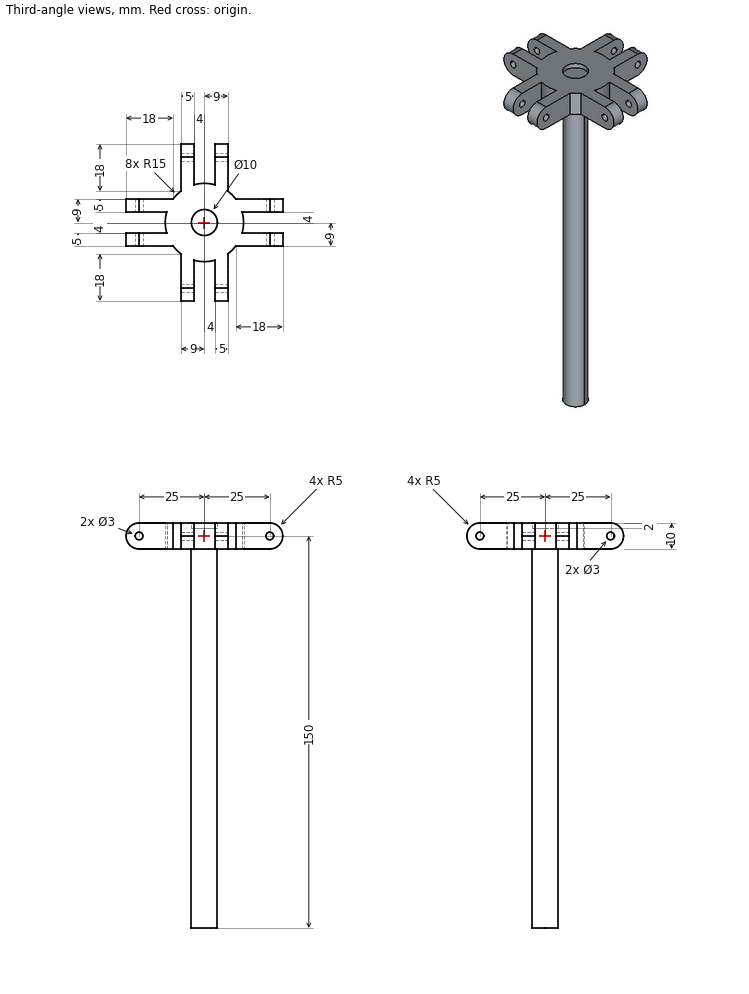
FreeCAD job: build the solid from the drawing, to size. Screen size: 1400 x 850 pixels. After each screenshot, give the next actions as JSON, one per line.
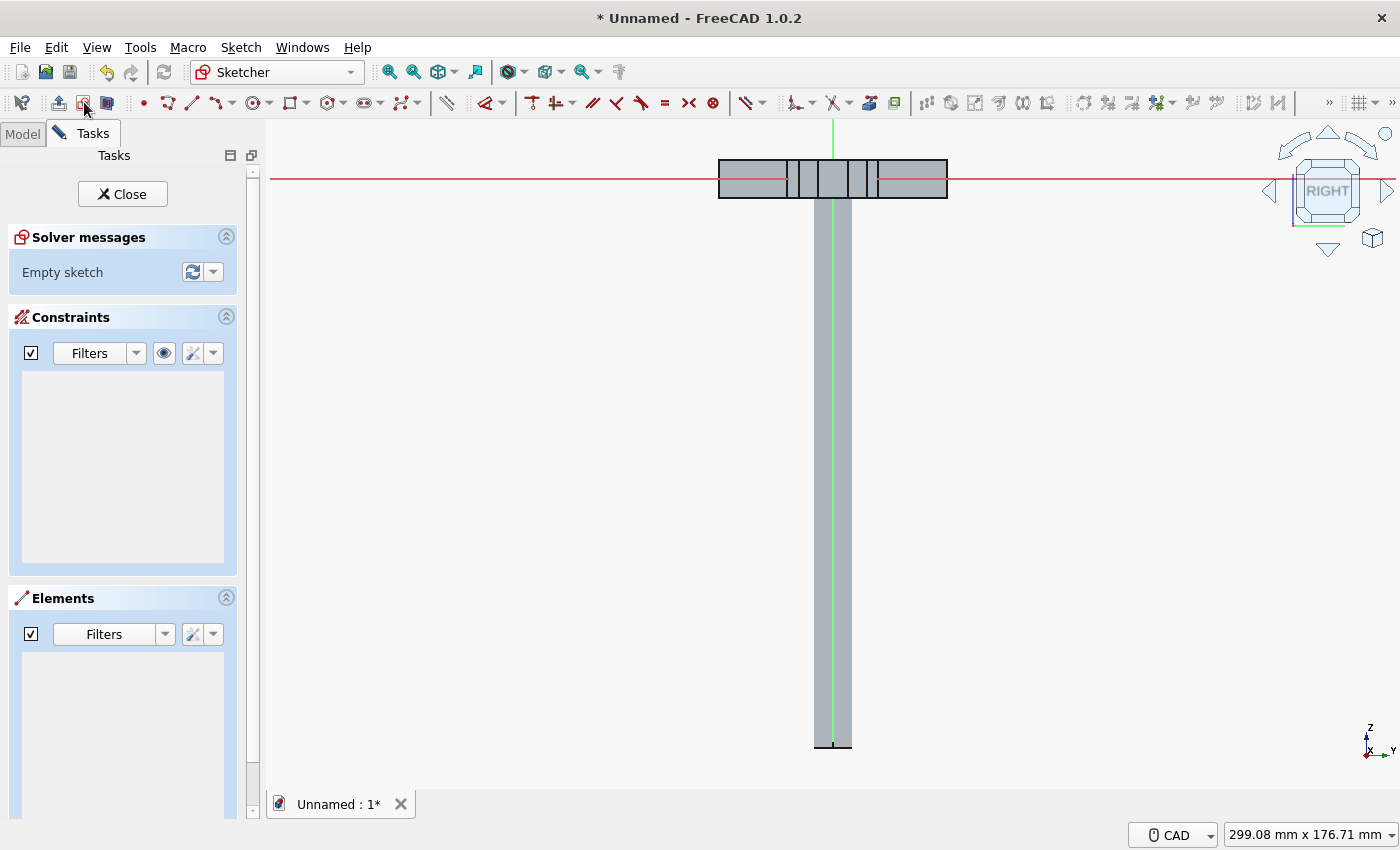
{"action": "scroll", "coordinate": [873, 147], "scroll_direction": "up", "scroll_amount": 5}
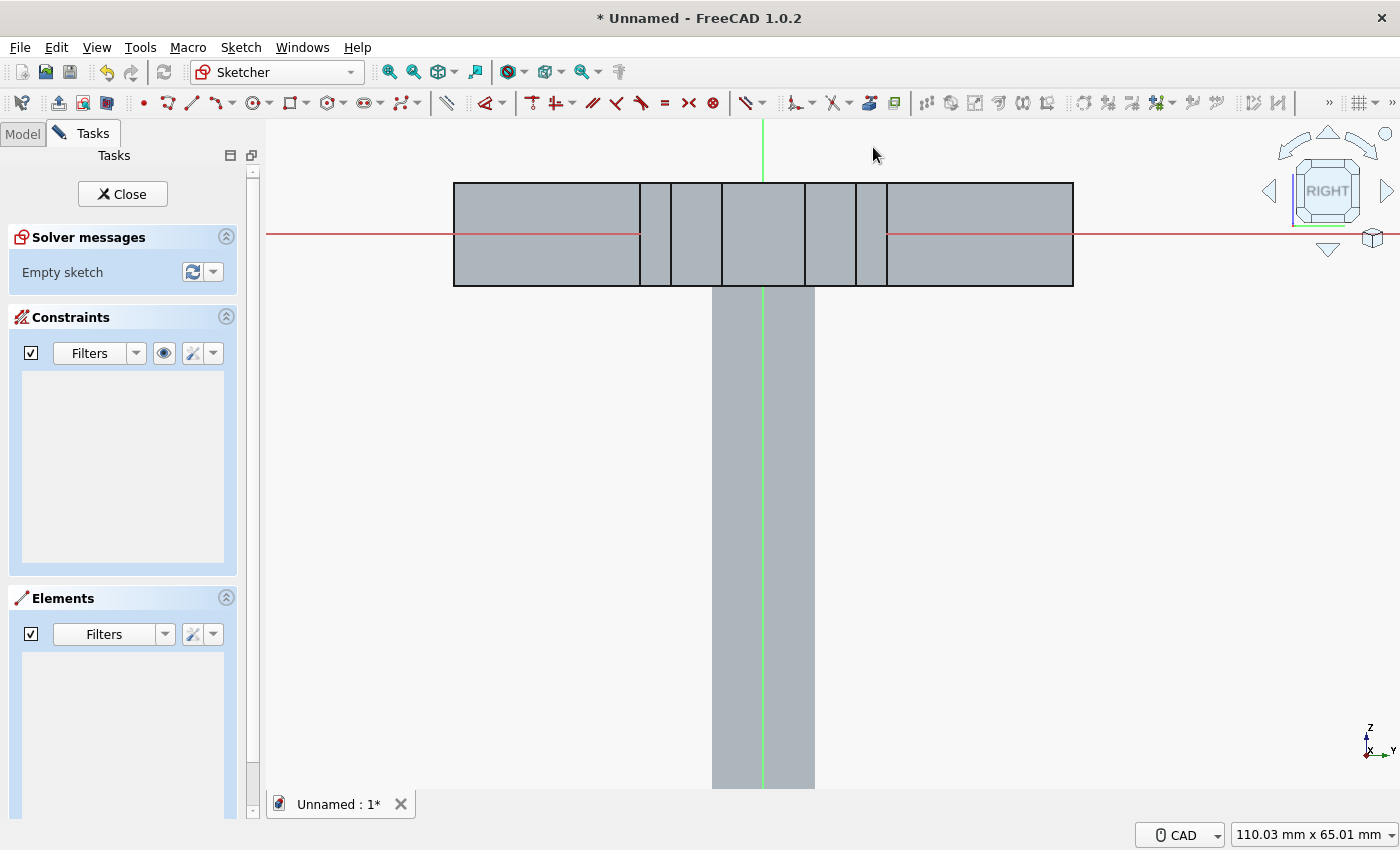
{"action": "left_click", "coordinate": [168, 104]}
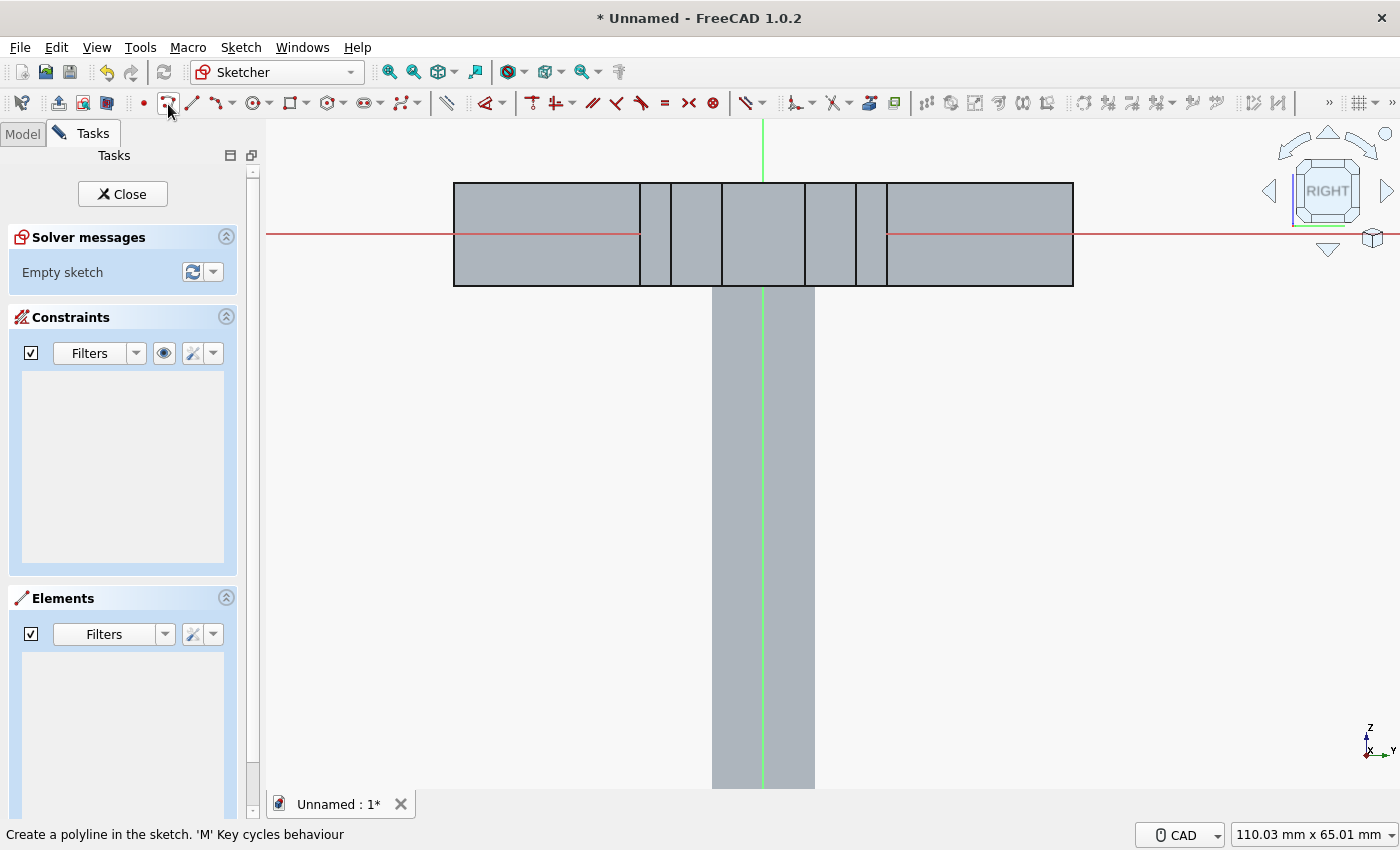
{"action": "left_click", "coordinate": [506, 183]}
{"action": "left_click", "coordinate": [454, 183]}
{"action": "left_click", "coordinate": [454, 234]}
{"action": "right_click", "coordinate": [454, 234]}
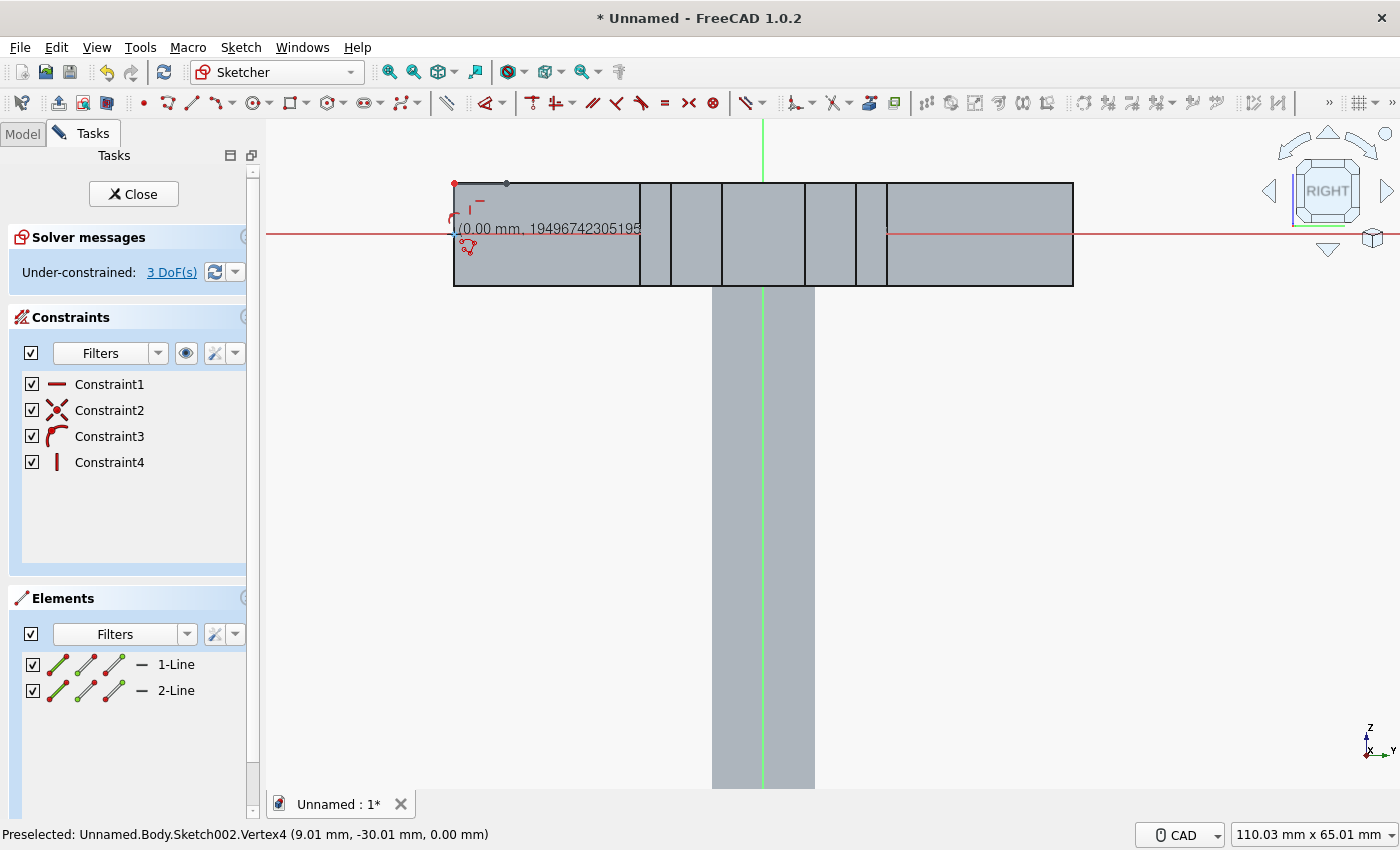
{"action": "key", "text": "g 3 a"}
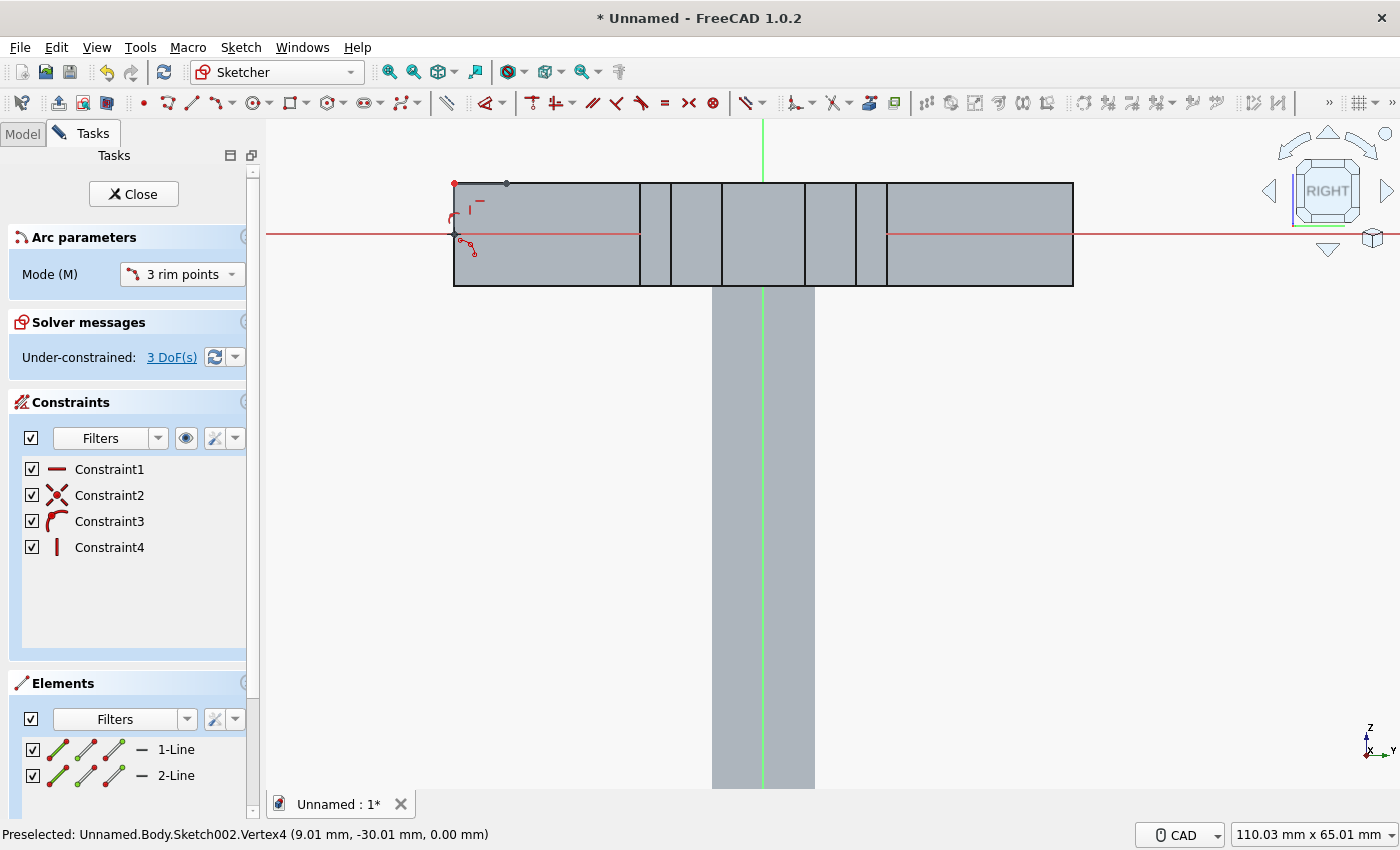
{"action": "left_click", "coordinate": [454, 234]}
{"action": "left_click", "coordinate": [506, 184]}
{"action": "left_click", "coordinate": [469, 198]}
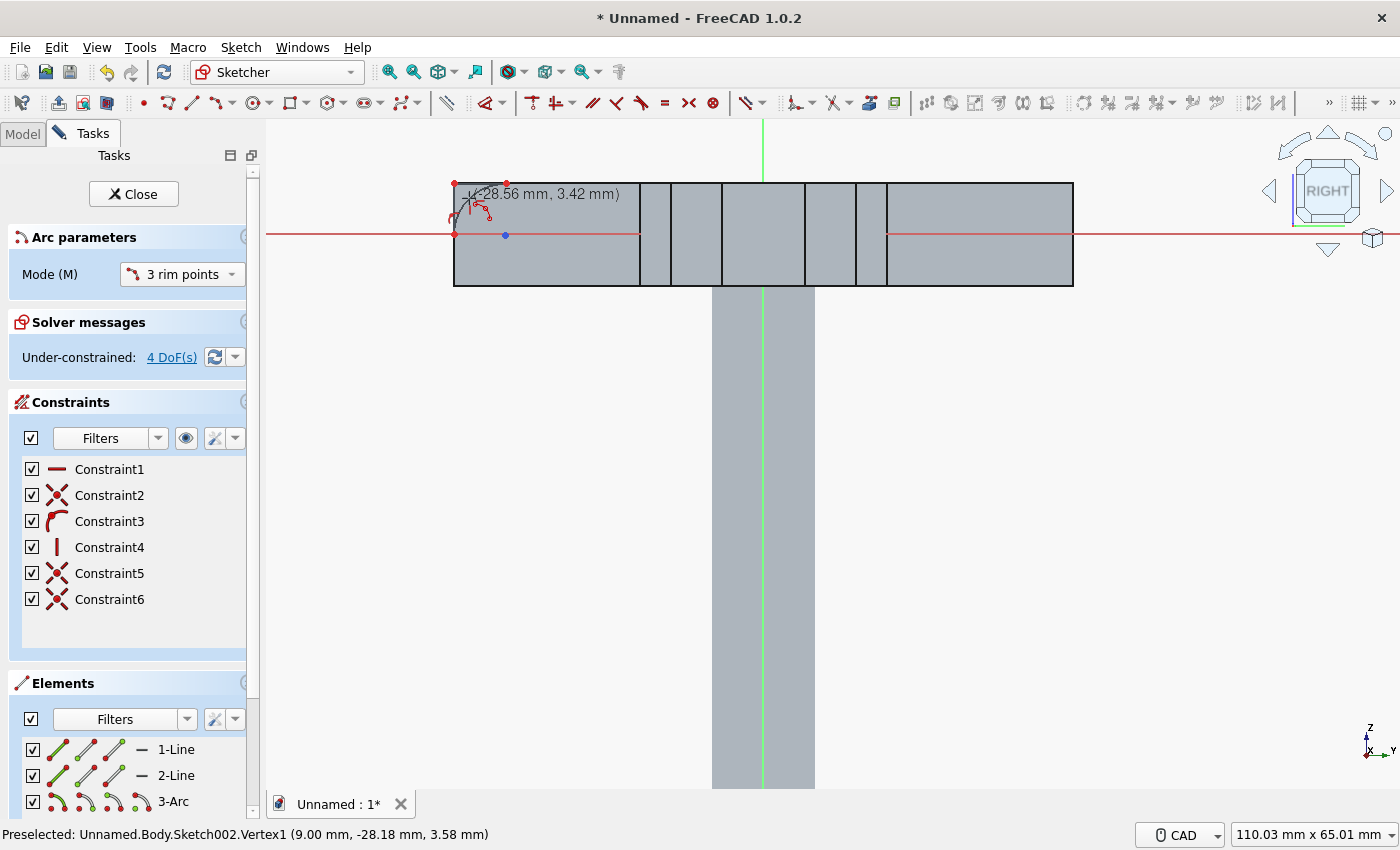
{"action": "left_click", "coordinate": [168, 104]}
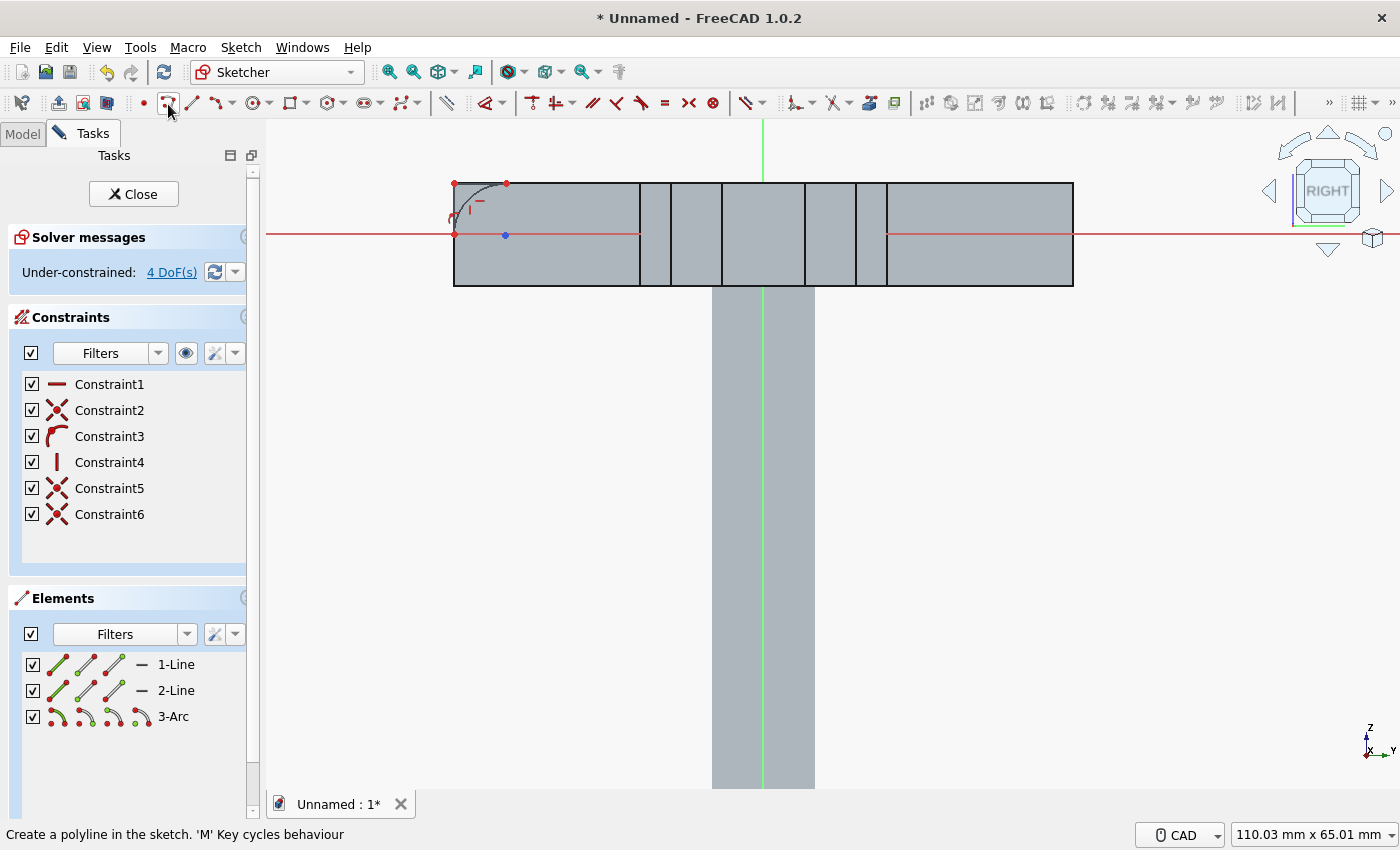
{"action": "left_click", "coordinate": [454, 234]}
{"action": "left_click", "coordinate": [454, 286]}
{"action": "left_click", "coordinate": [506, 286]}
{"action": "right_click", "coordinate": [506, 286]}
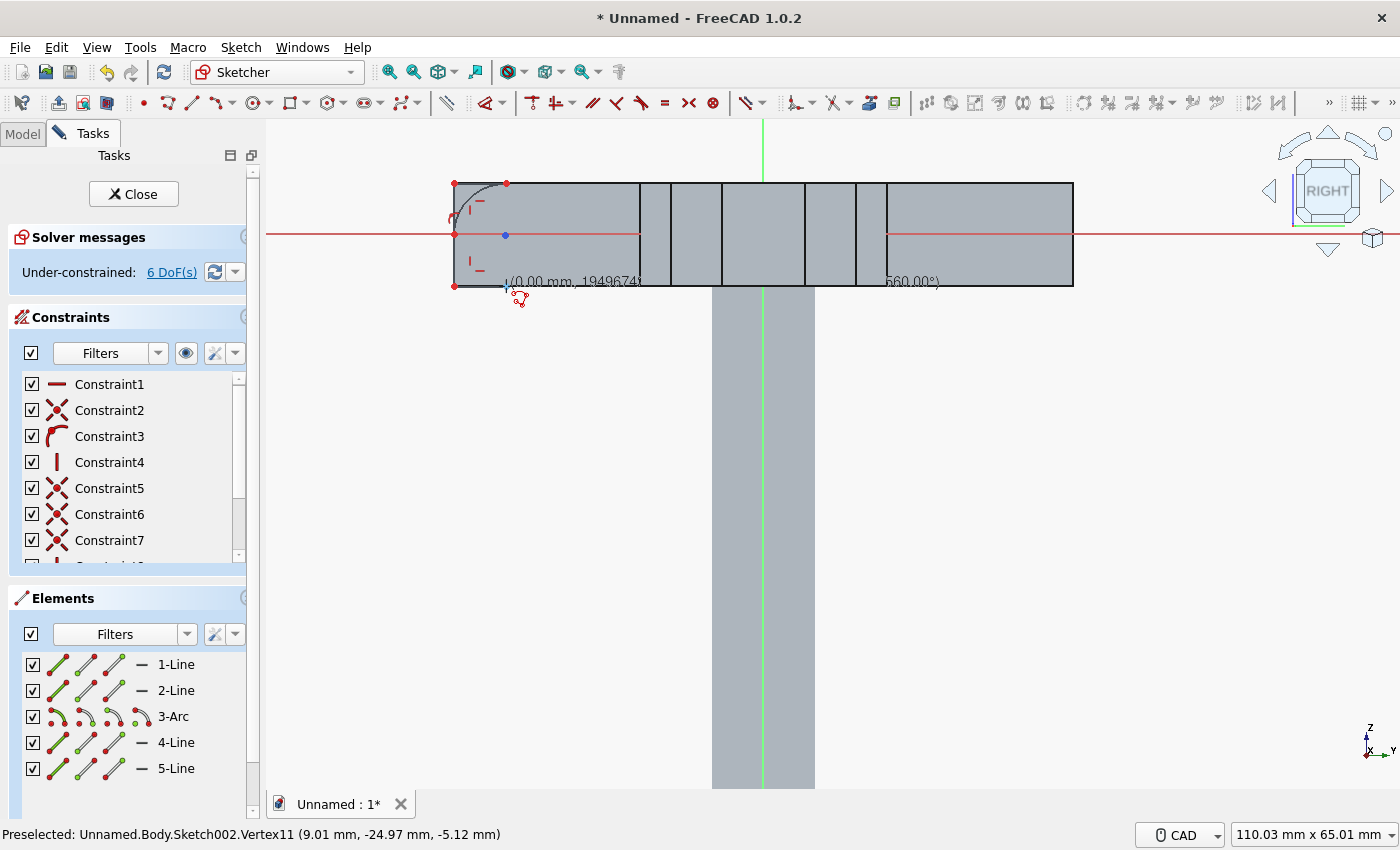
{"action": "key", "text": "g 3 a"}